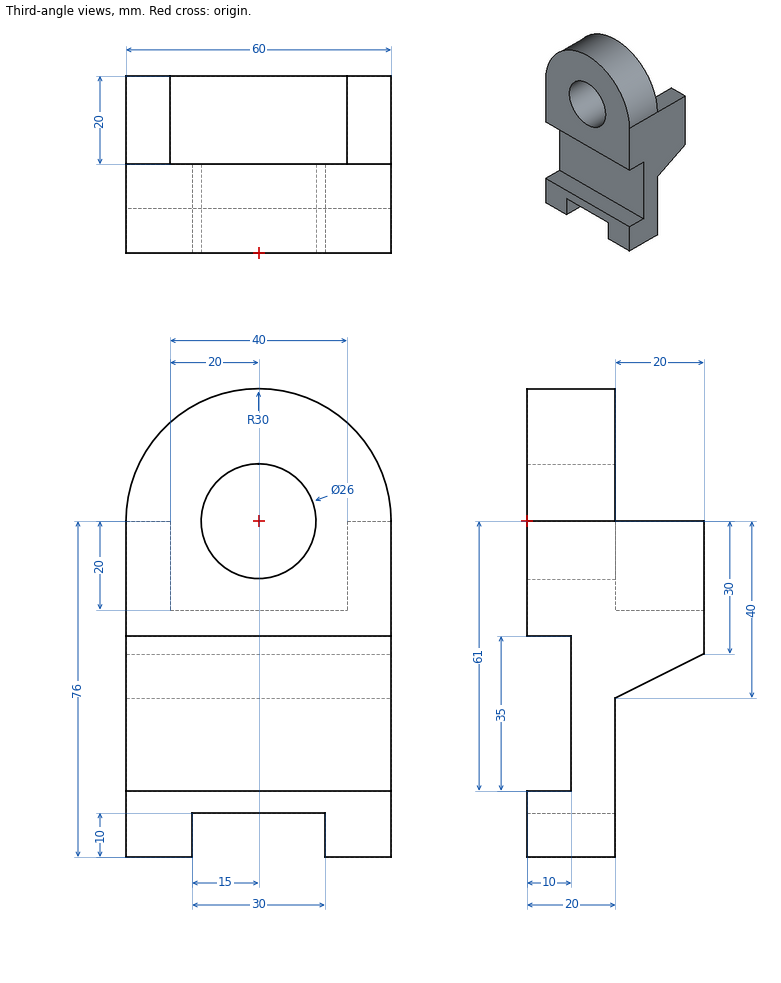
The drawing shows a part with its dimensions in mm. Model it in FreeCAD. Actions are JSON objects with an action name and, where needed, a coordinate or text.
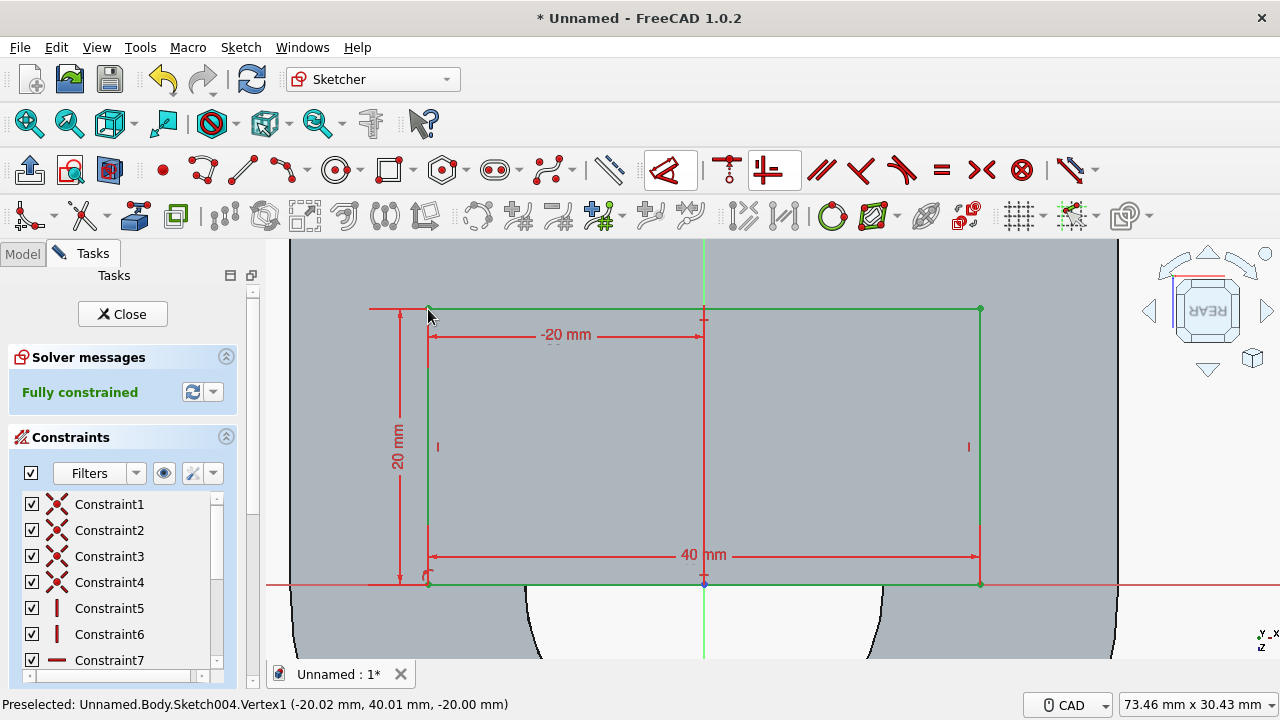
{"action": "left_click", "coordinate": [123, 314]}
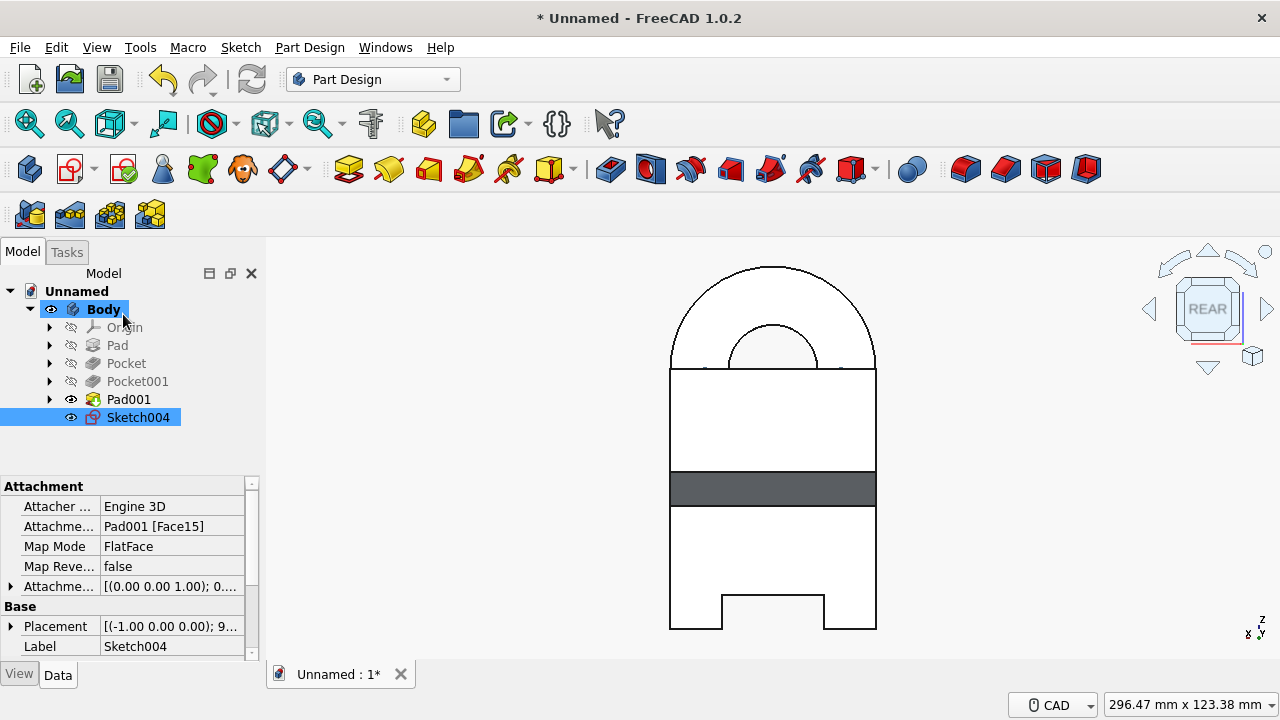
{"action": "left_click", "coordinate": [612, 170]}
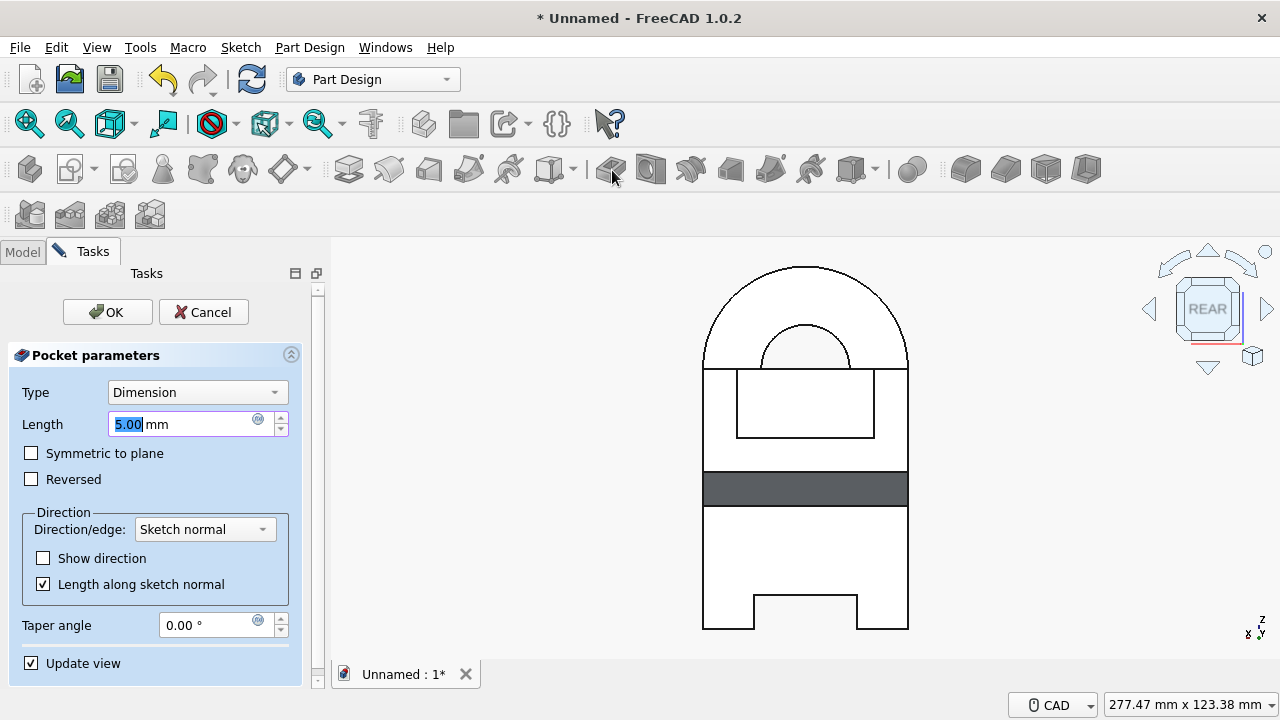
{"action": "type", "text": "20"}
{"action": "key", "text": "Tab"}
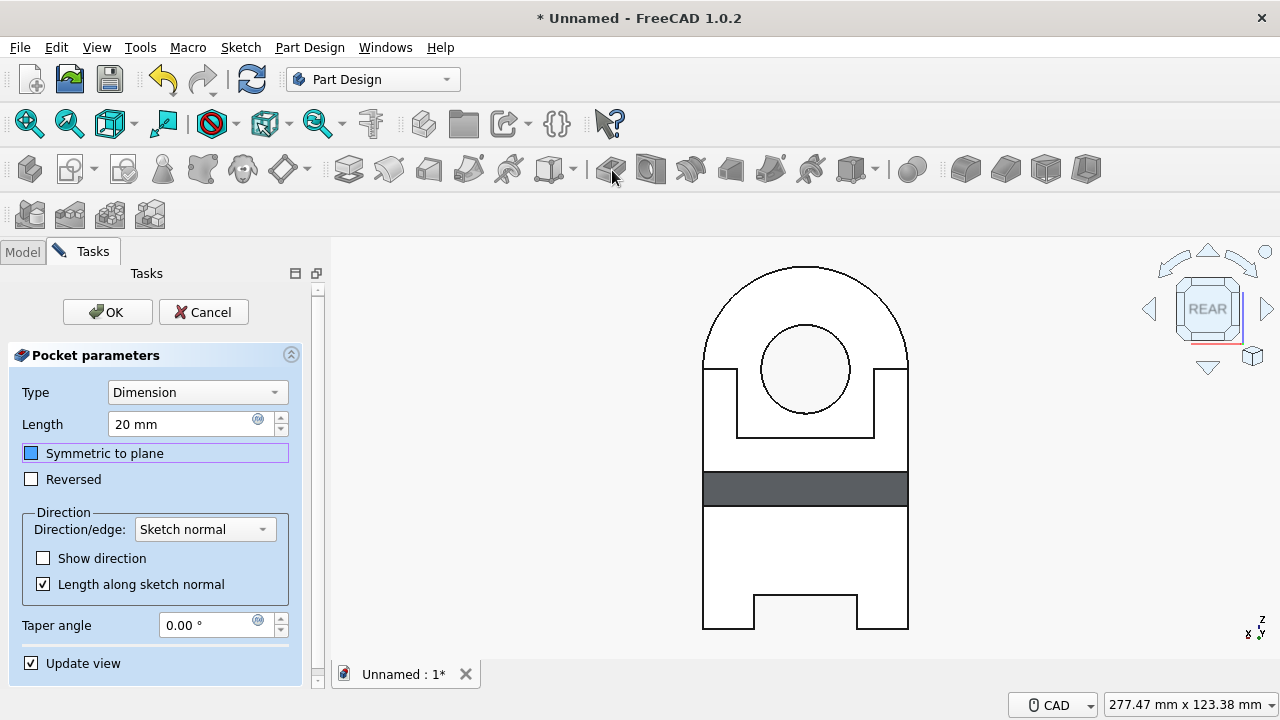
{"action": "left_click", "coordinate": [108, 312]}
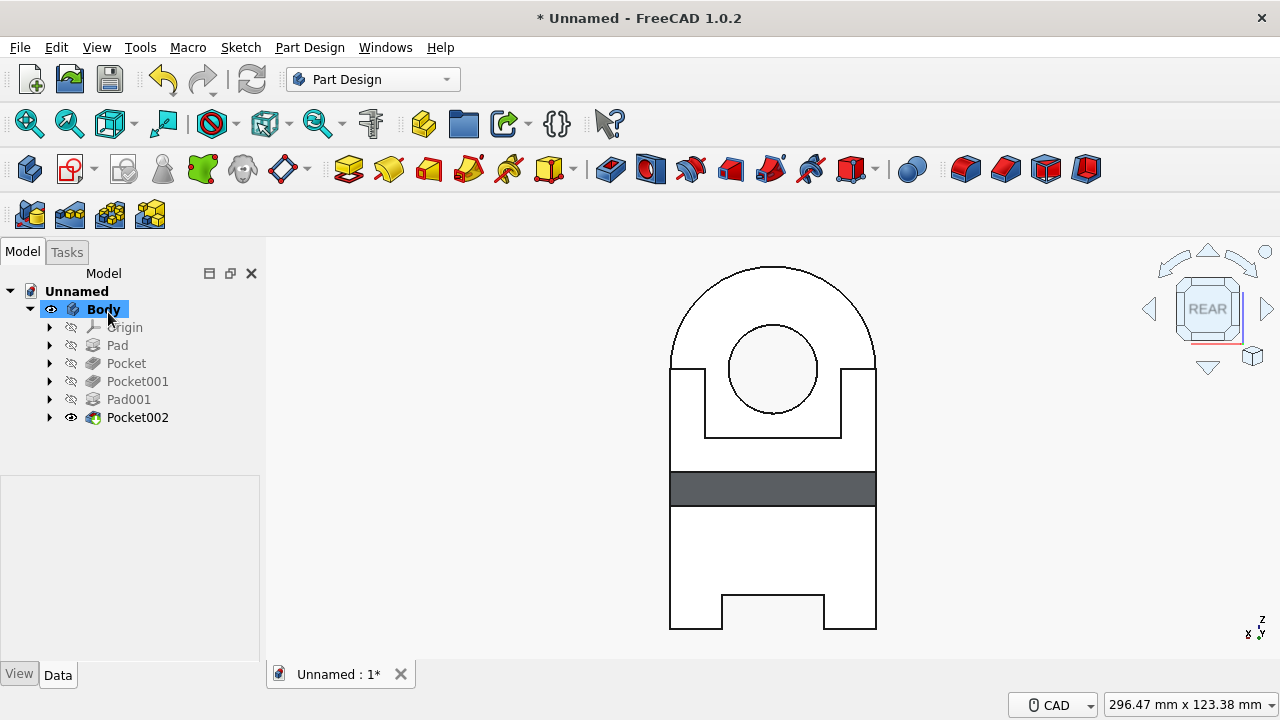
{"action": "key", "text": "0"}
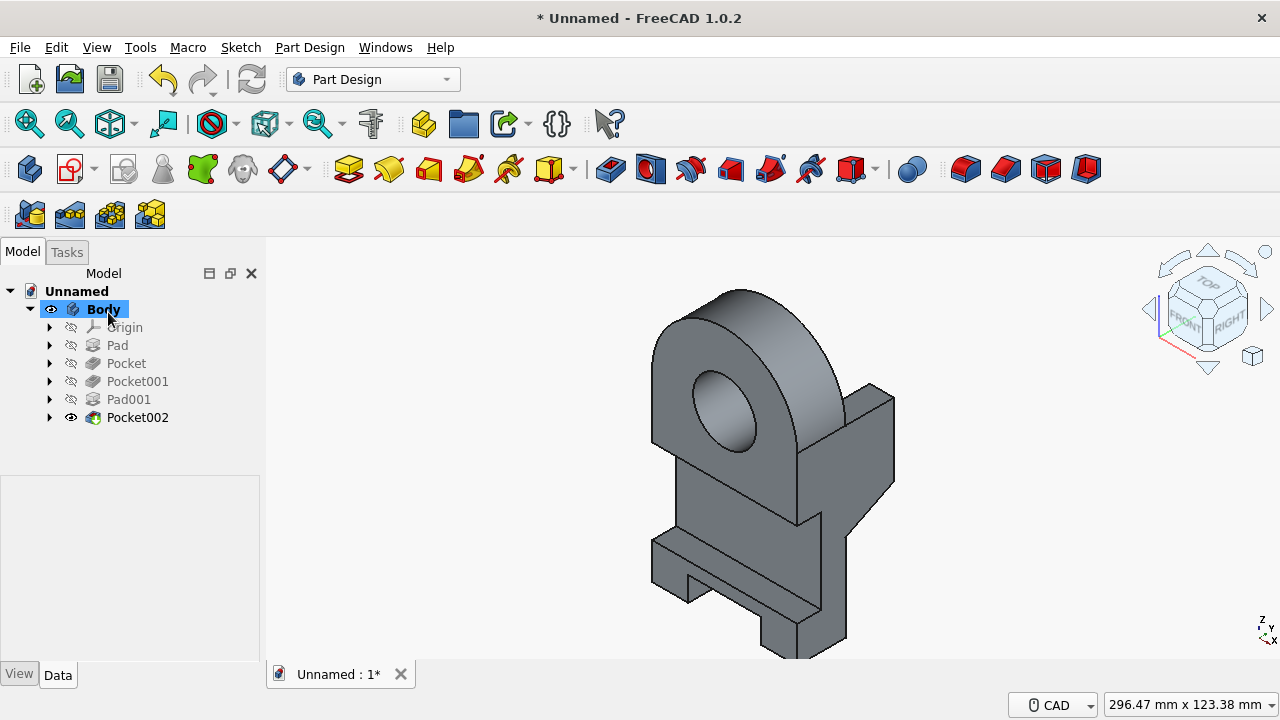
{"action": "key", "text": "v f"}